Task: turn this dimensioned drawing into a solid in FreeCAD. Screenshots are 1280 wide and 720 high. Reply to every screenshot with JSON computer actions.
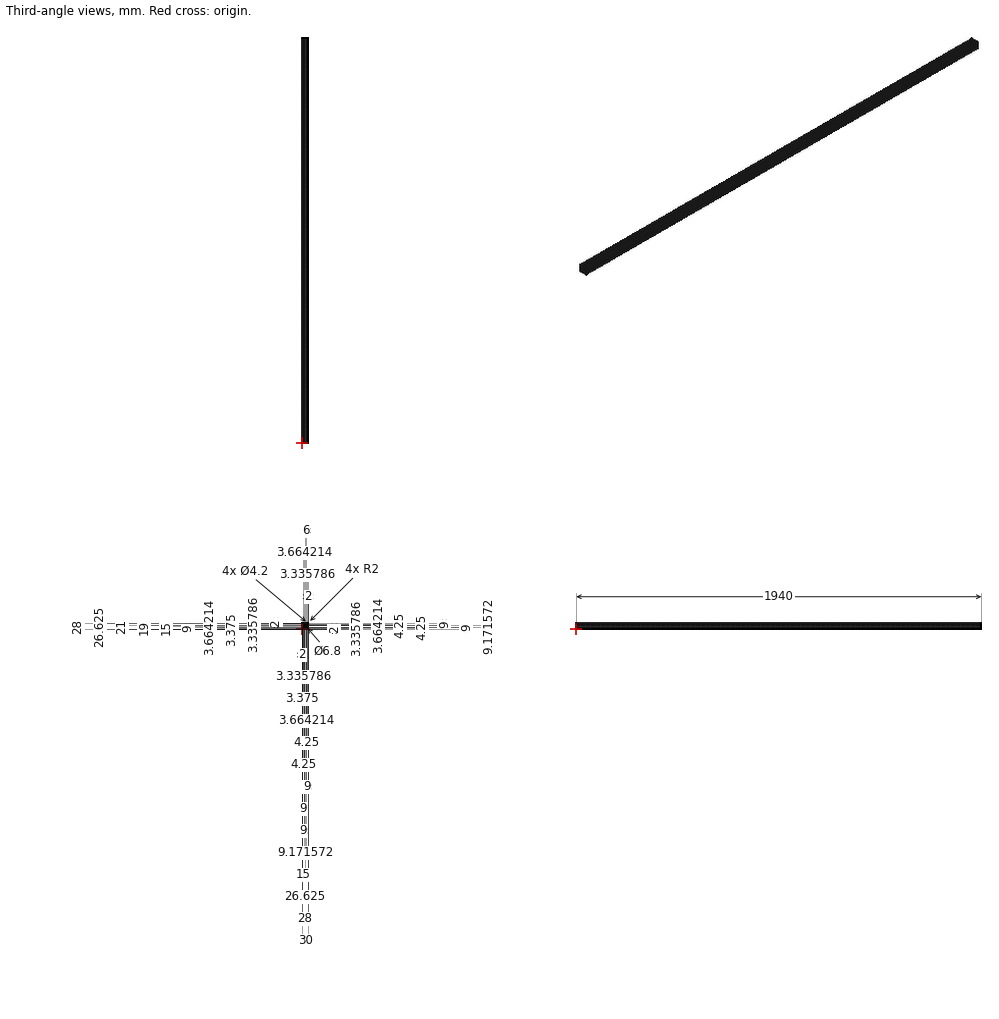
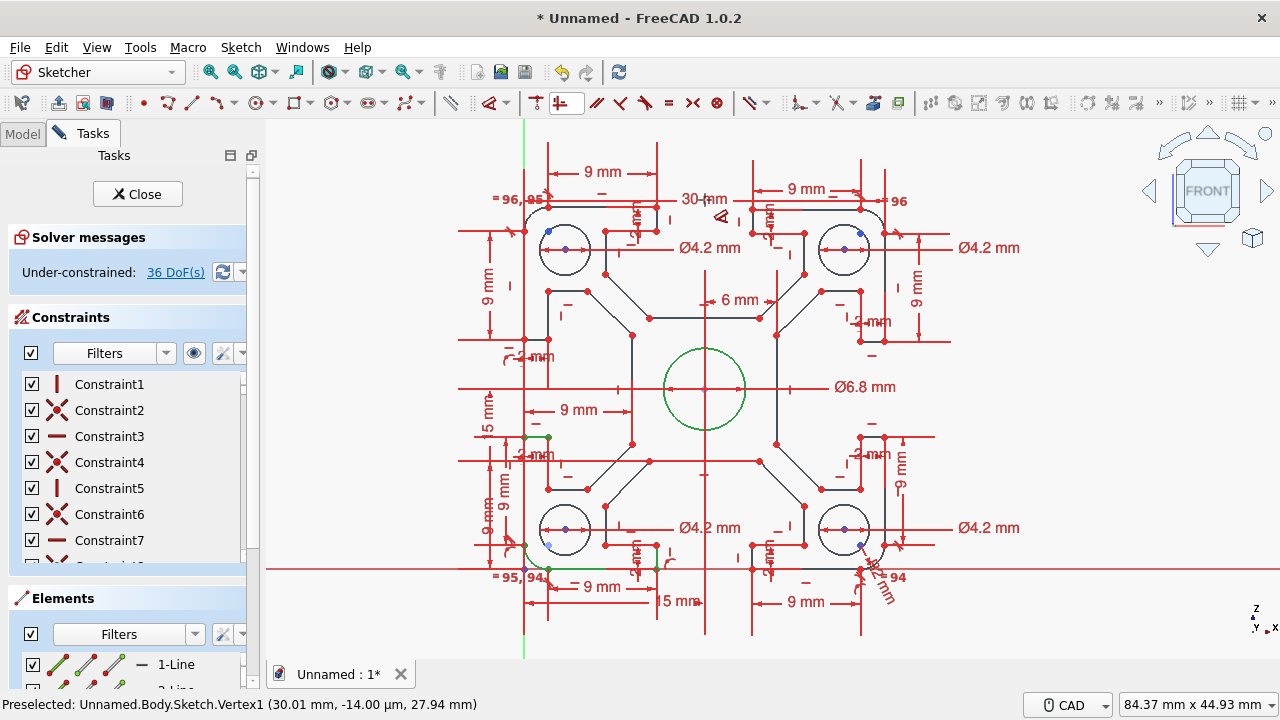
{"action": "left_click", "coordinate": [885, 234]}
{"action": "left_click", "coordinate": [919, 402]}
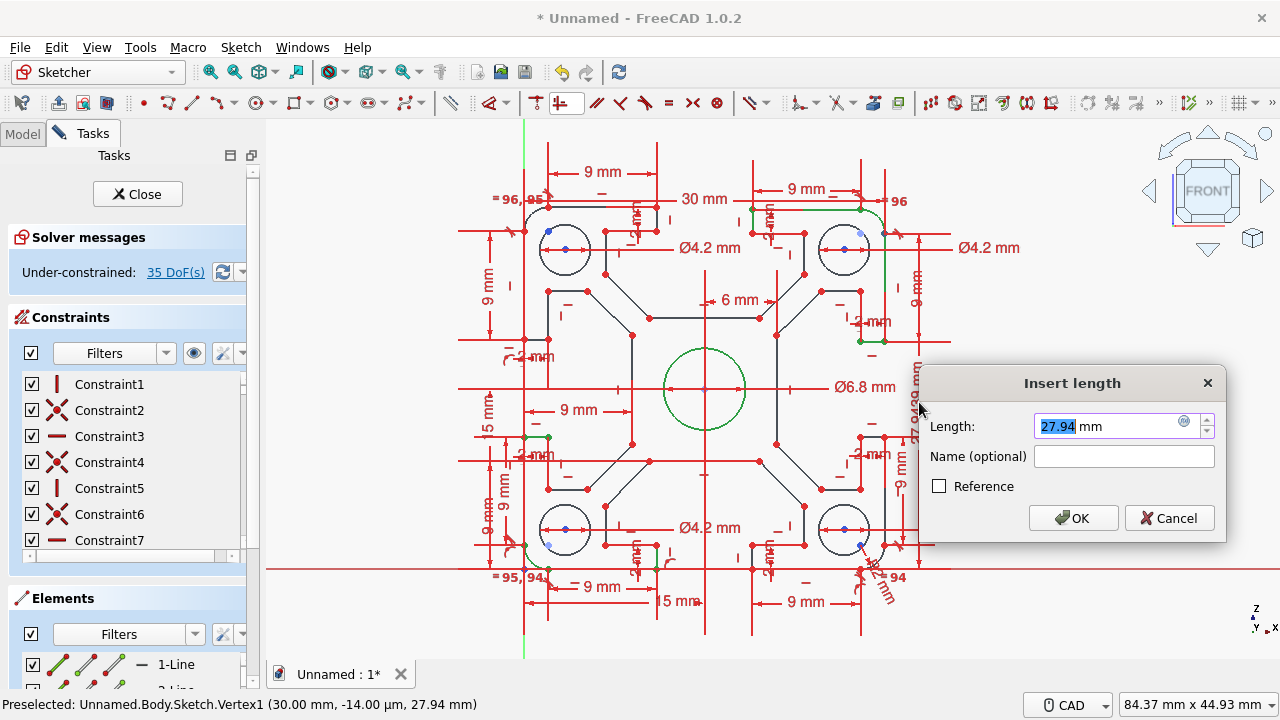
{"action": "type", "text": "28"}
{"action": "key", "text": "Return"}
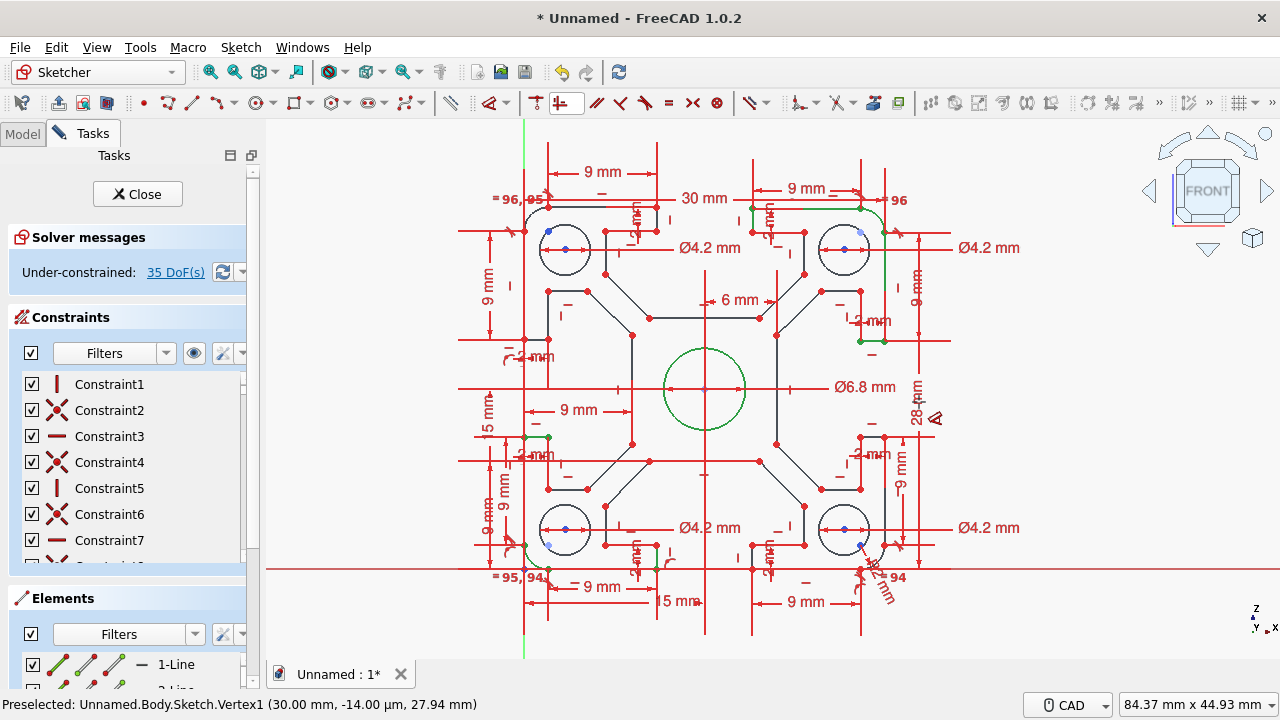
{"action": "left_click", "coordinate": [861, 490]}
{"action": "left_click", "coordinate": [692, 627]}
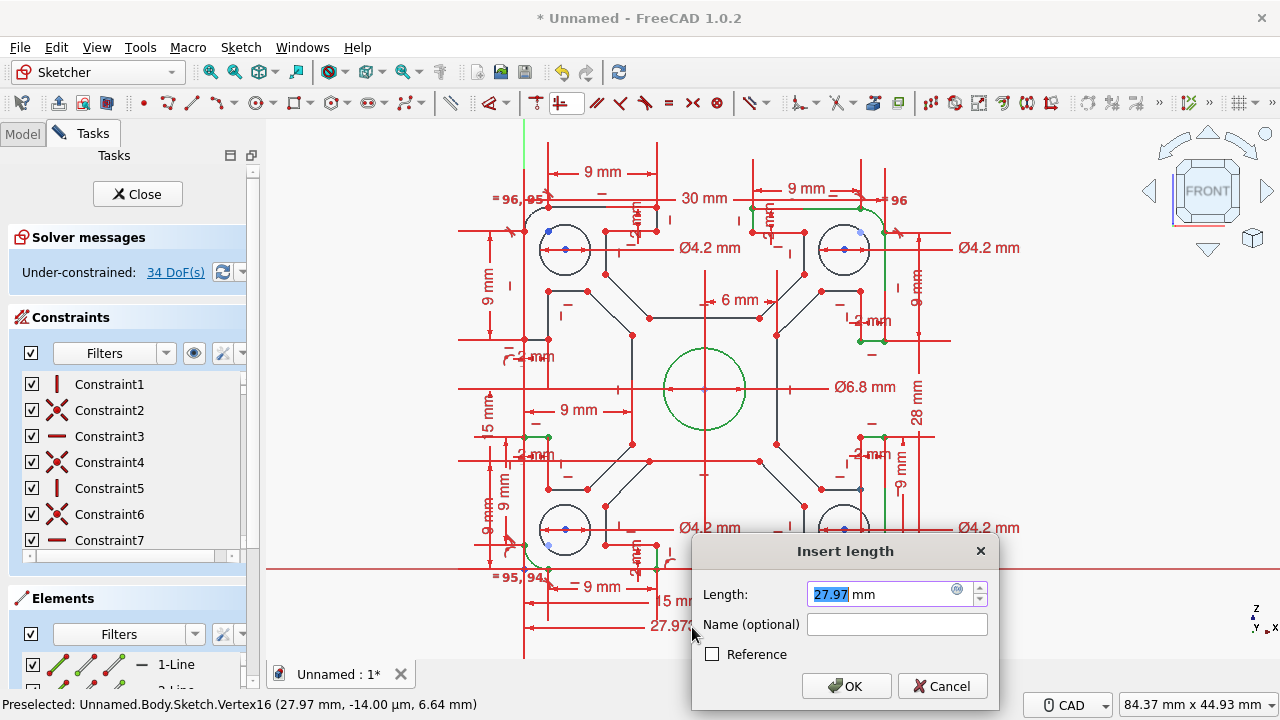
{"action": "type", "text": "28"}
{"action": "key", "text": "Return"}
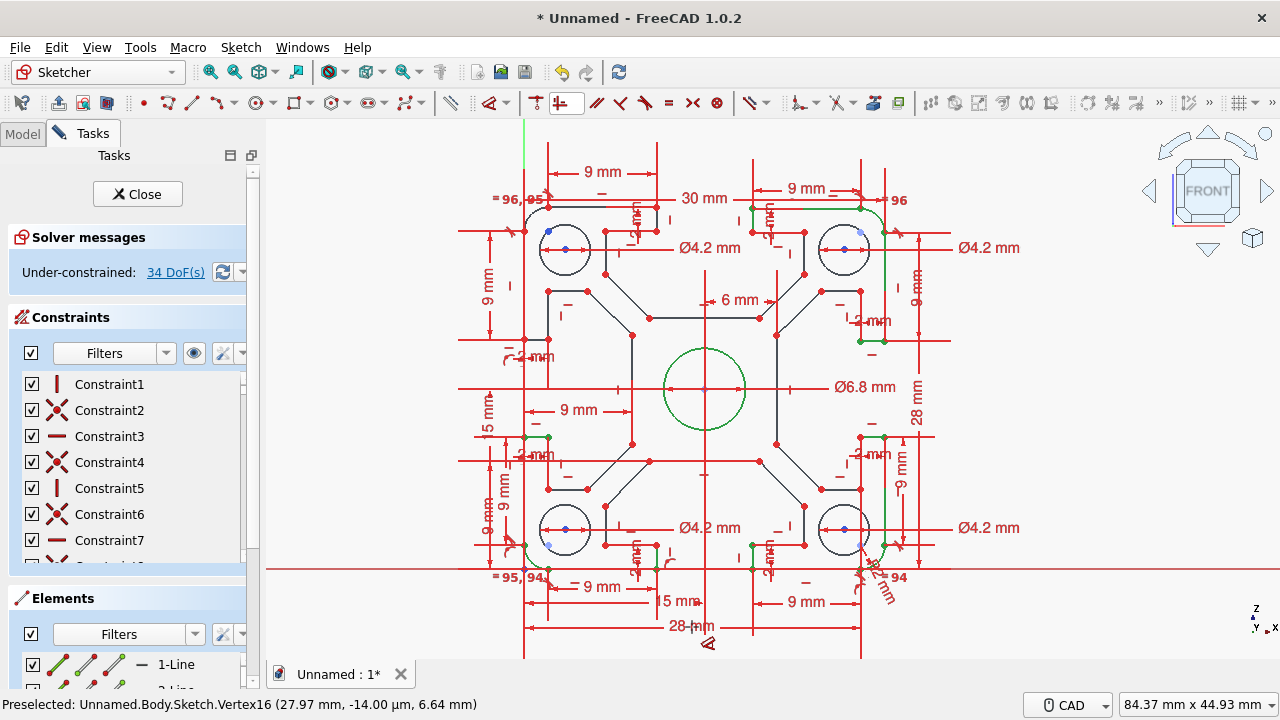
{"action": "left_click", "coordinate": [548, 340]}
{"action": "left_click", "coordinate": [606, 374]}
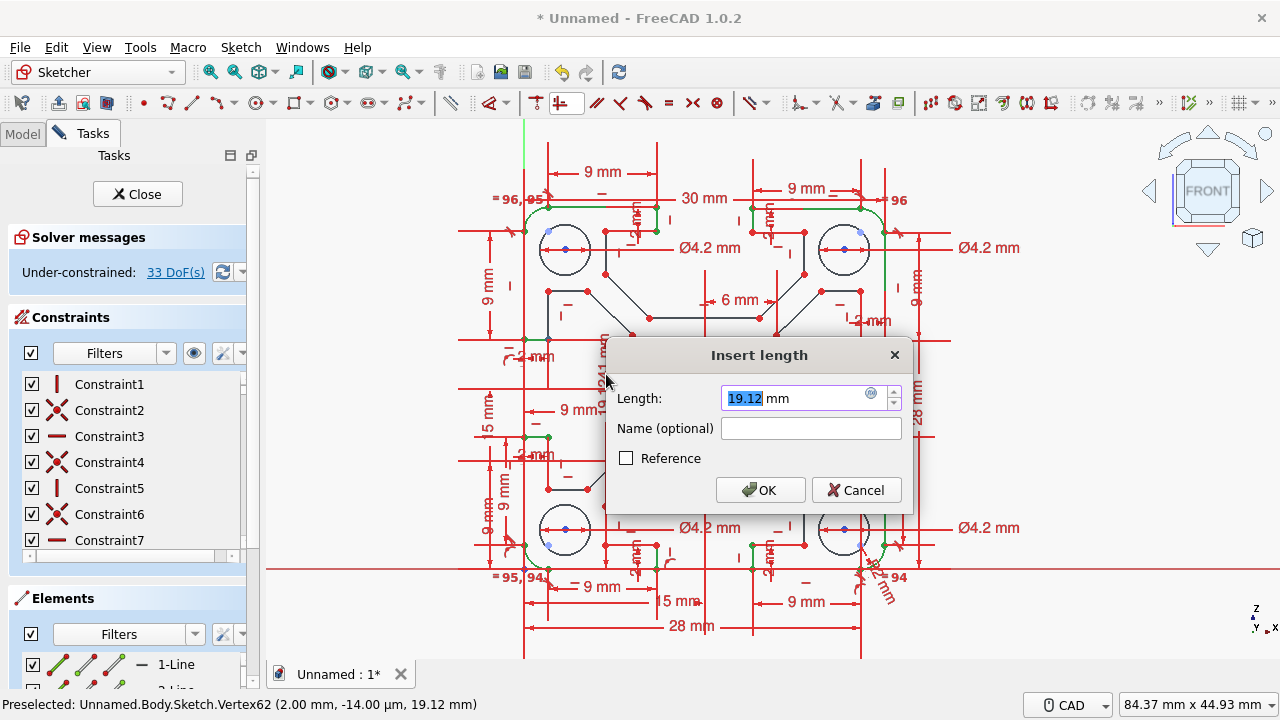
{"action": "type", "text": "19"}
{"action": "key", "text": "Return"}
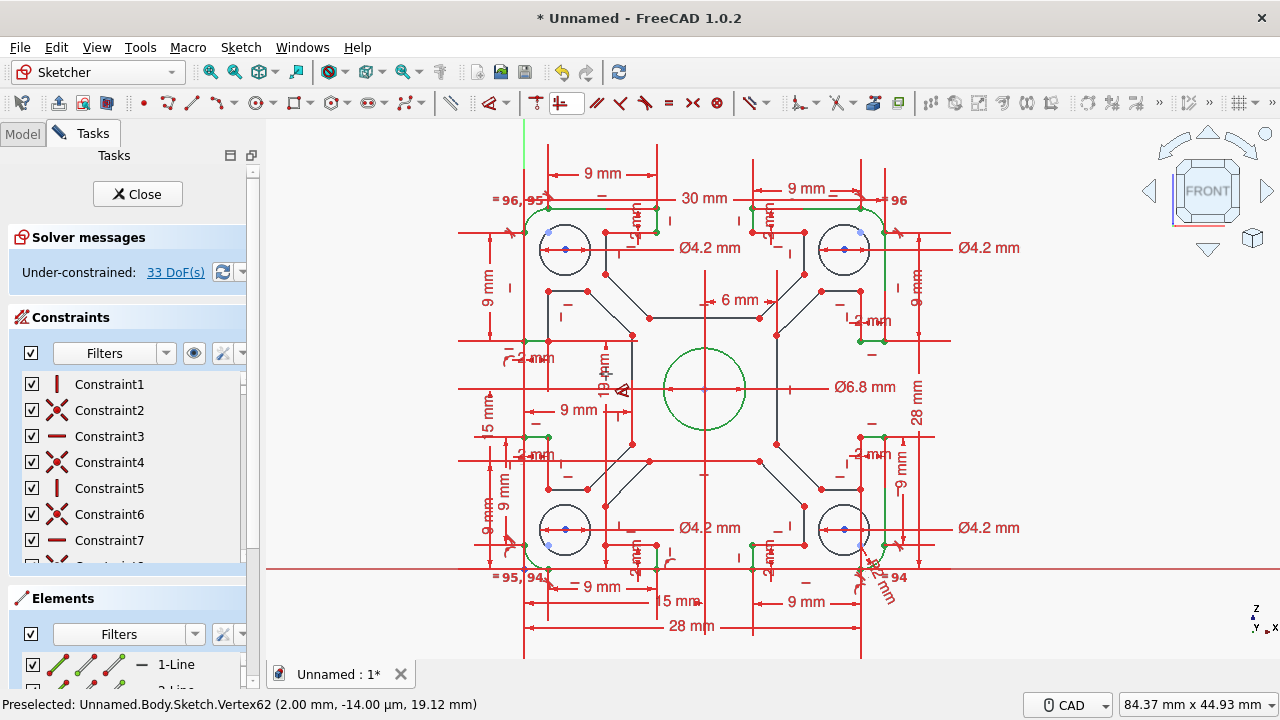
{"action": "left_click", "coordinate": [650, 318]}
{"action": "left_click", "coordinate": [490, 386]}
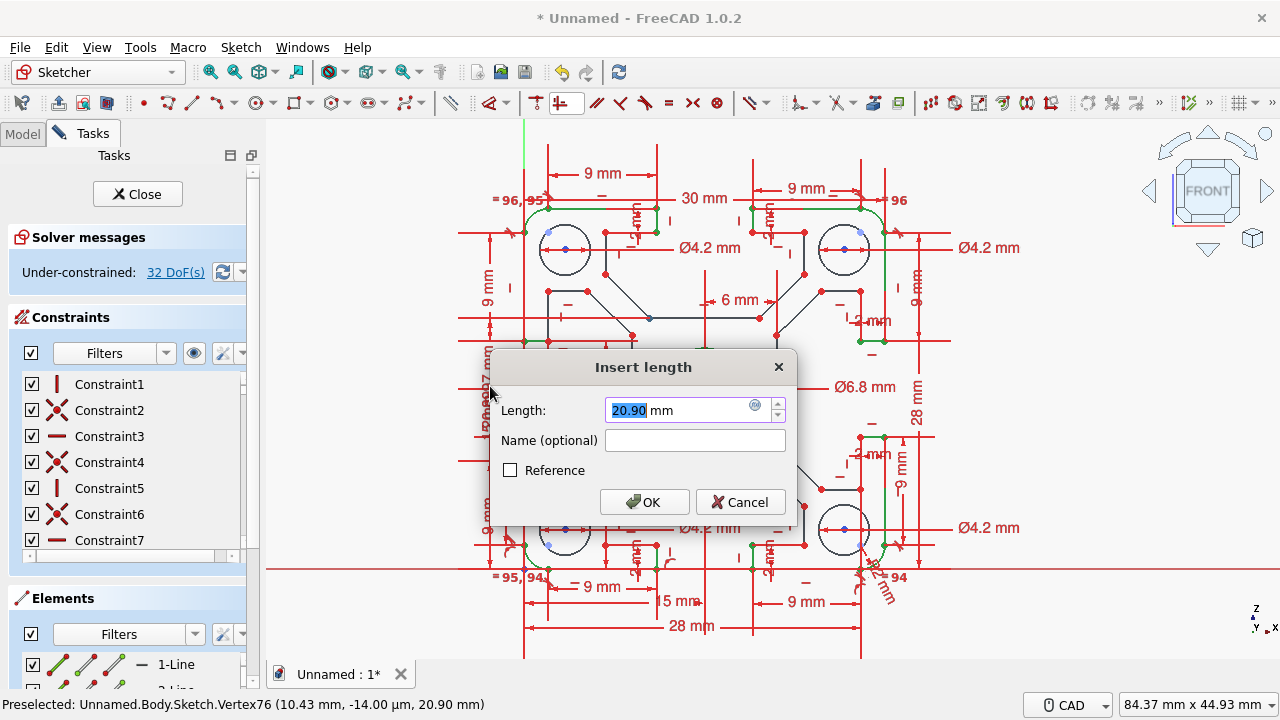
{"action": "type", "text": "21"}
{"action": "key", "text": "Return"}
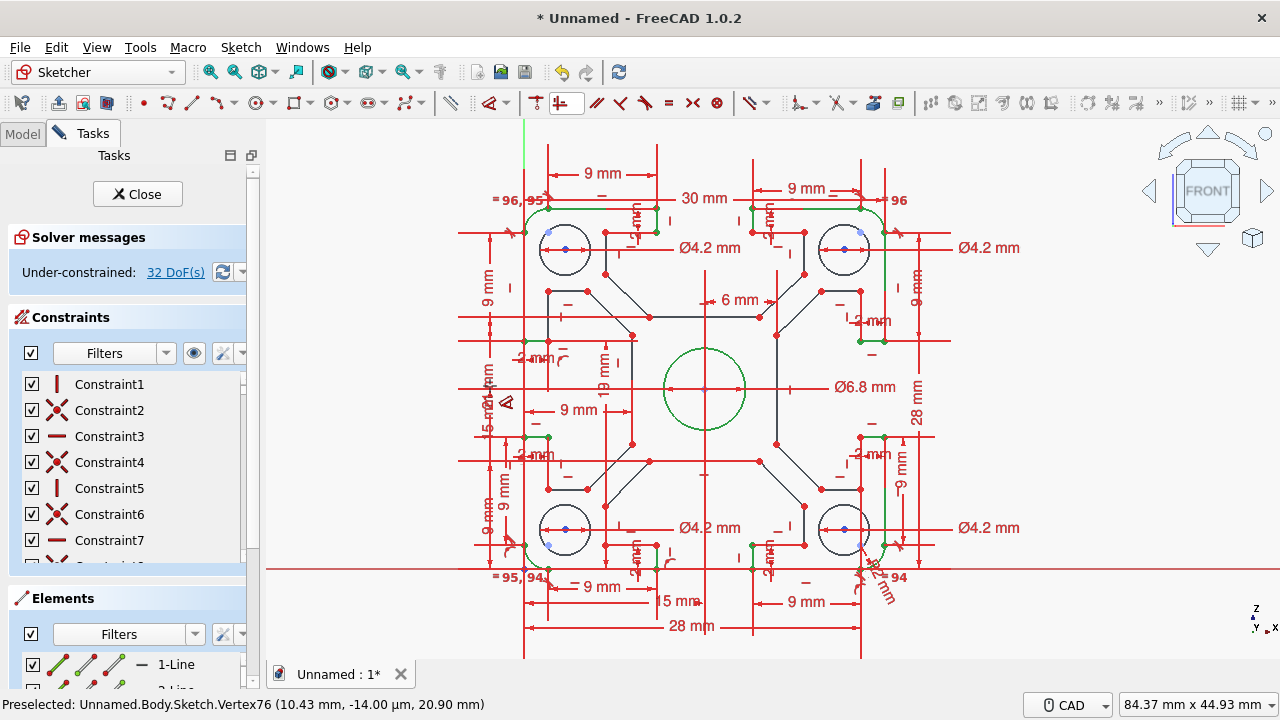
{"action": "left_click", "coordinate": [861, 326]}
{"action": "left_click", "coordinate": [803, 334]}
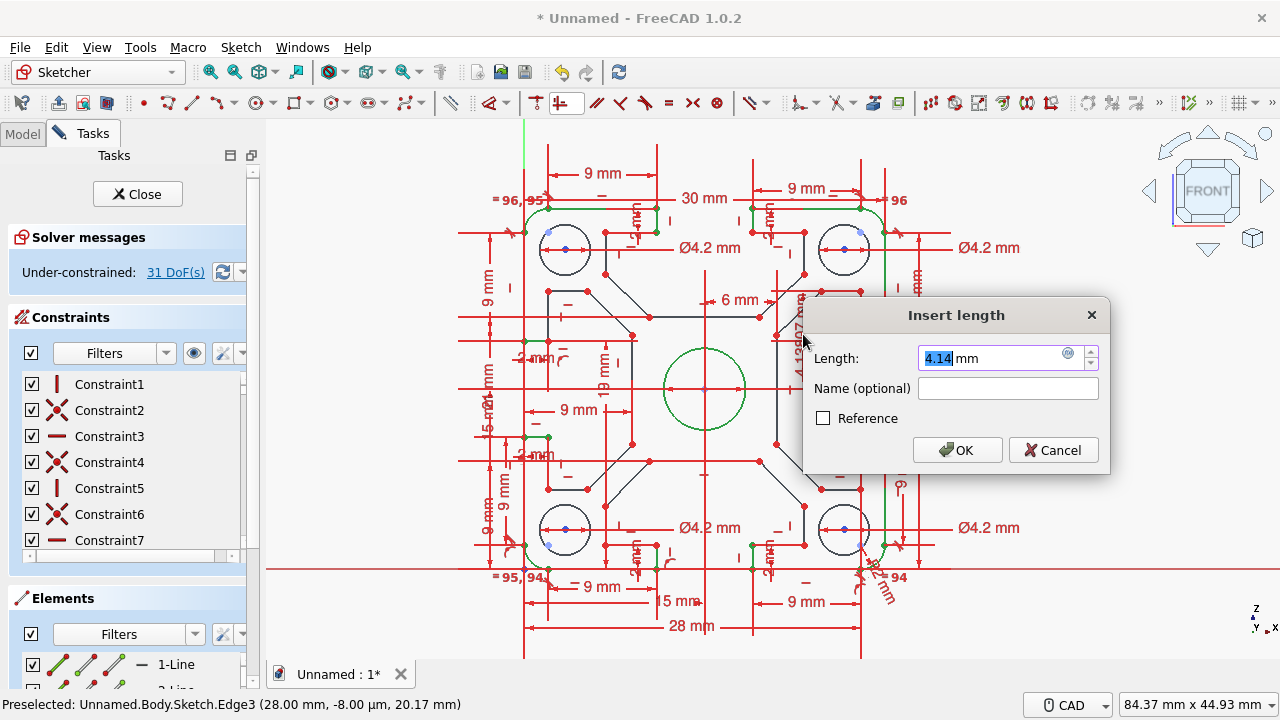
{"action": "type", "text": "4.25"}
{"action": "key", "text": "Return"}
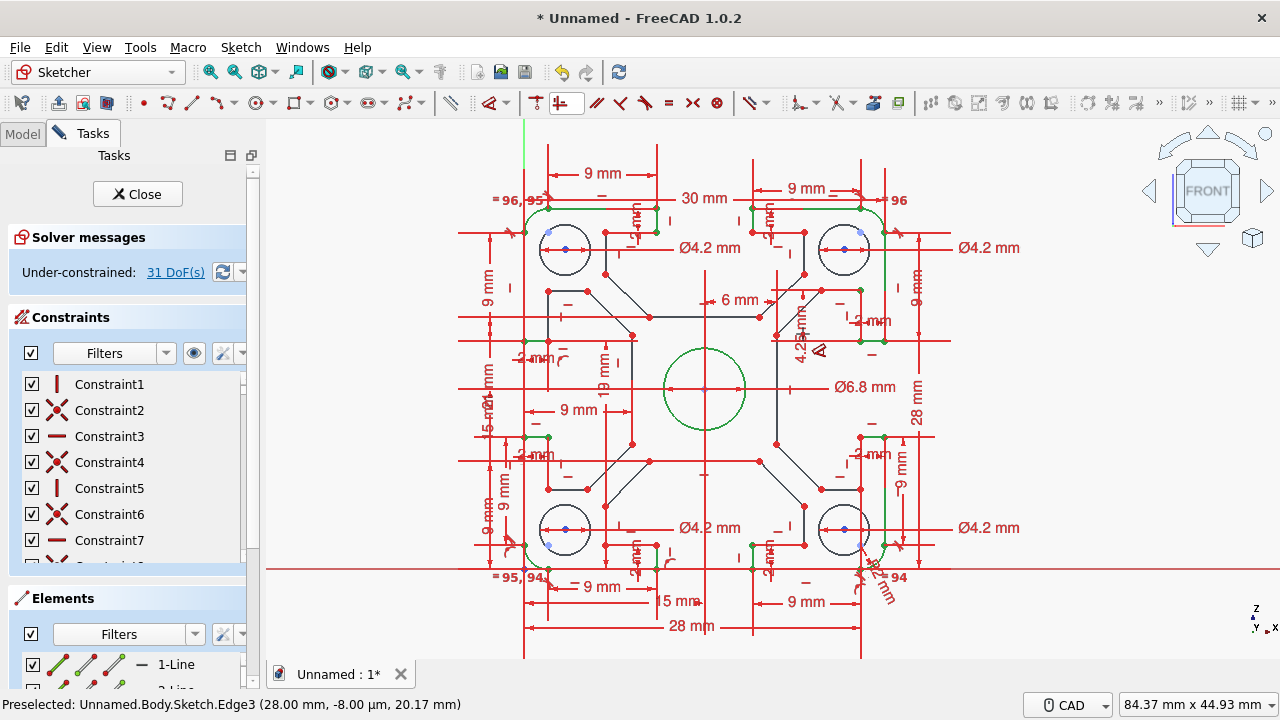
{"action": "left_click", "coordinate": [861, 474]}
{"action": "left_click", "coordinate": [943, 445]}